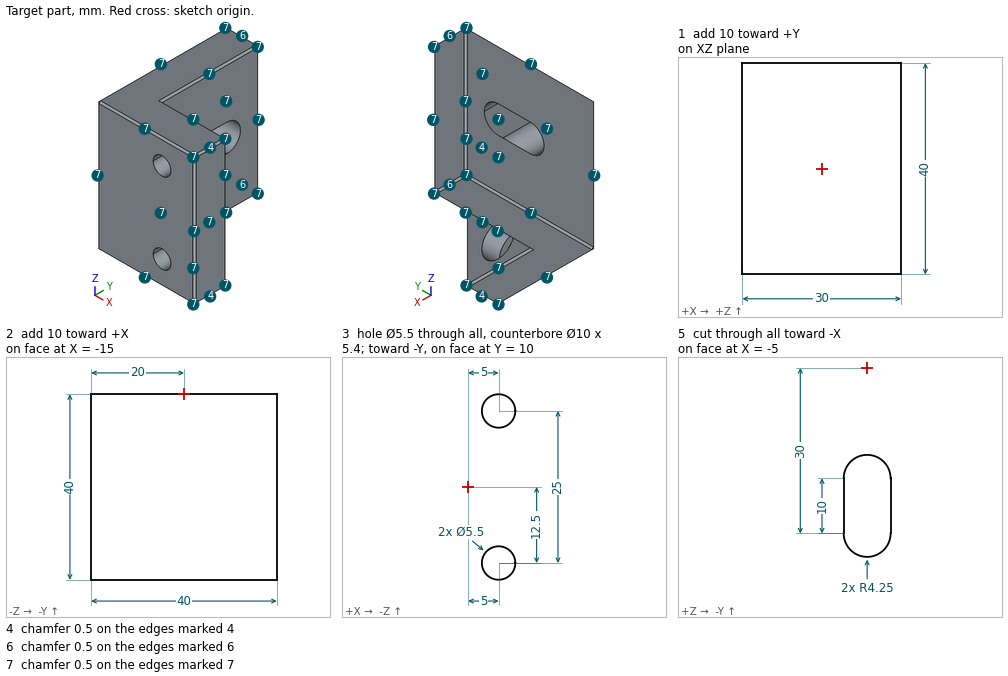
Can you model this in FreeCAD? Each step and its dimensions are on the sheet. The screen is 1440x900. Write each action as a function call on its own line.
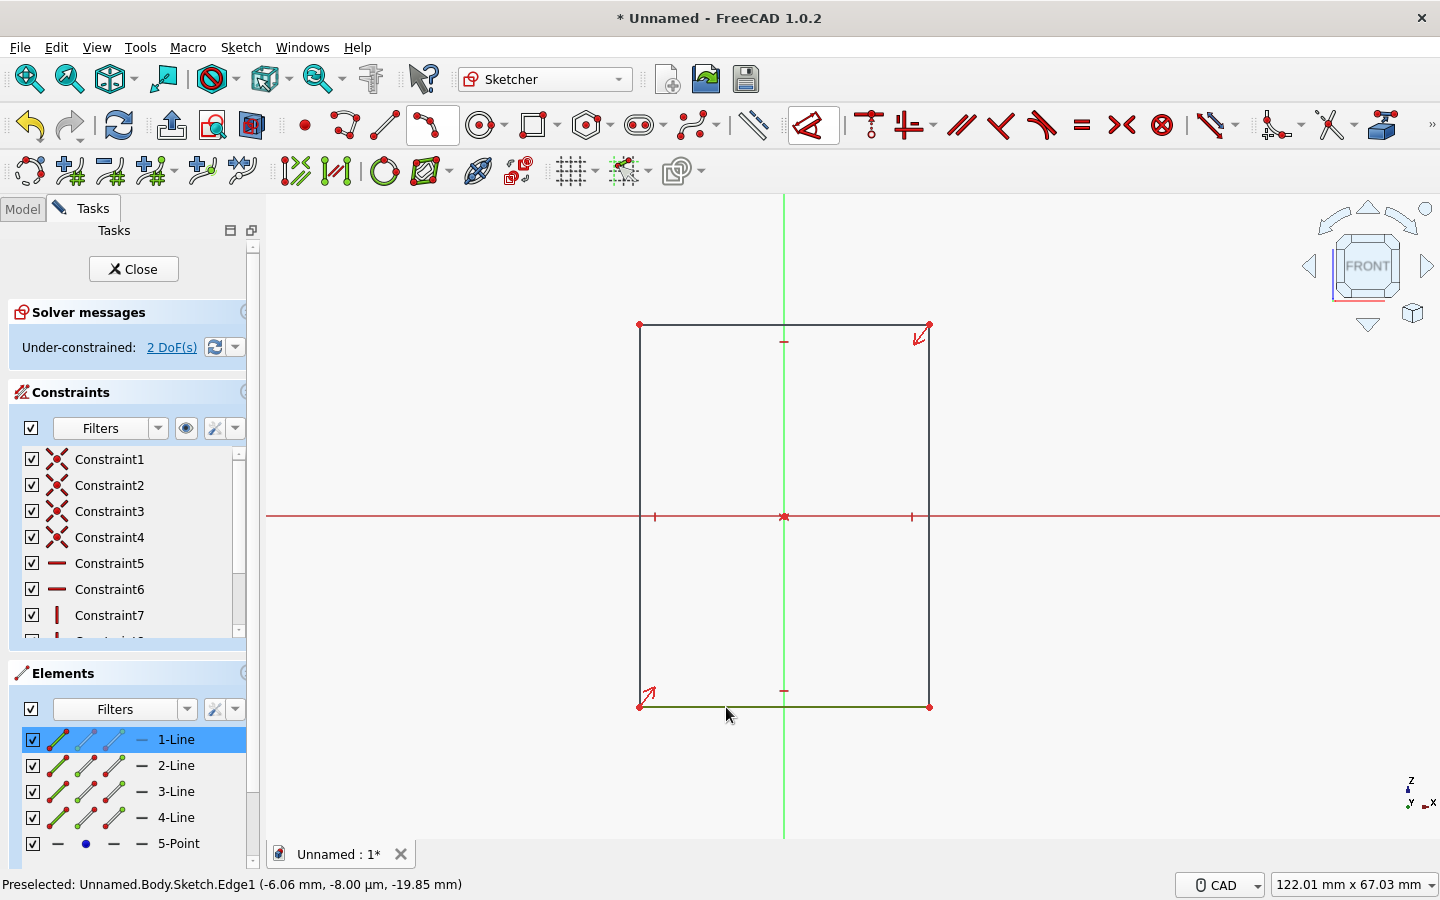
click(834, 126)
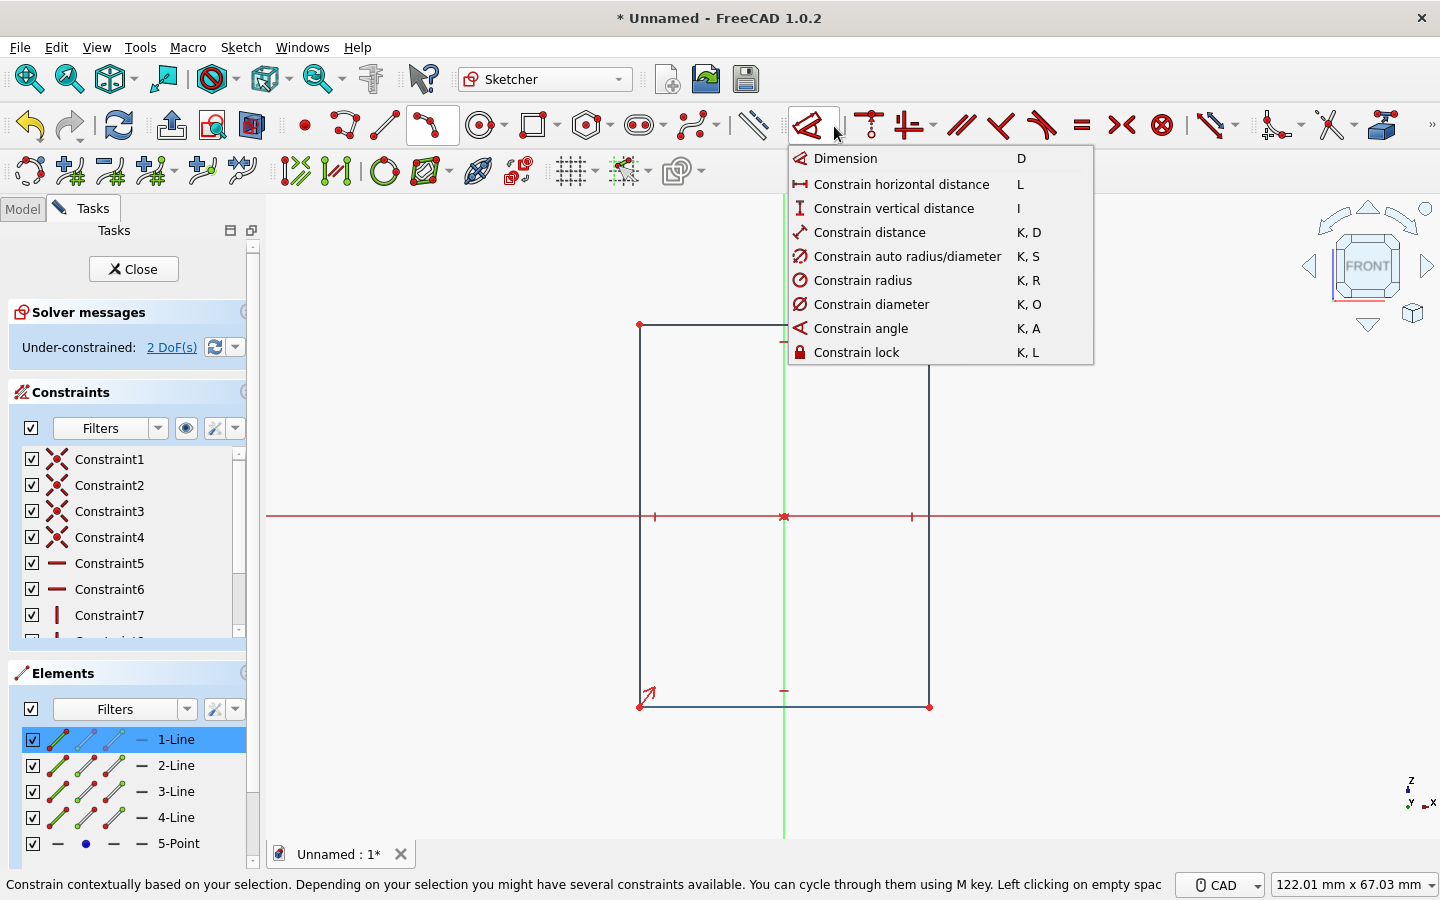
click(941, 184)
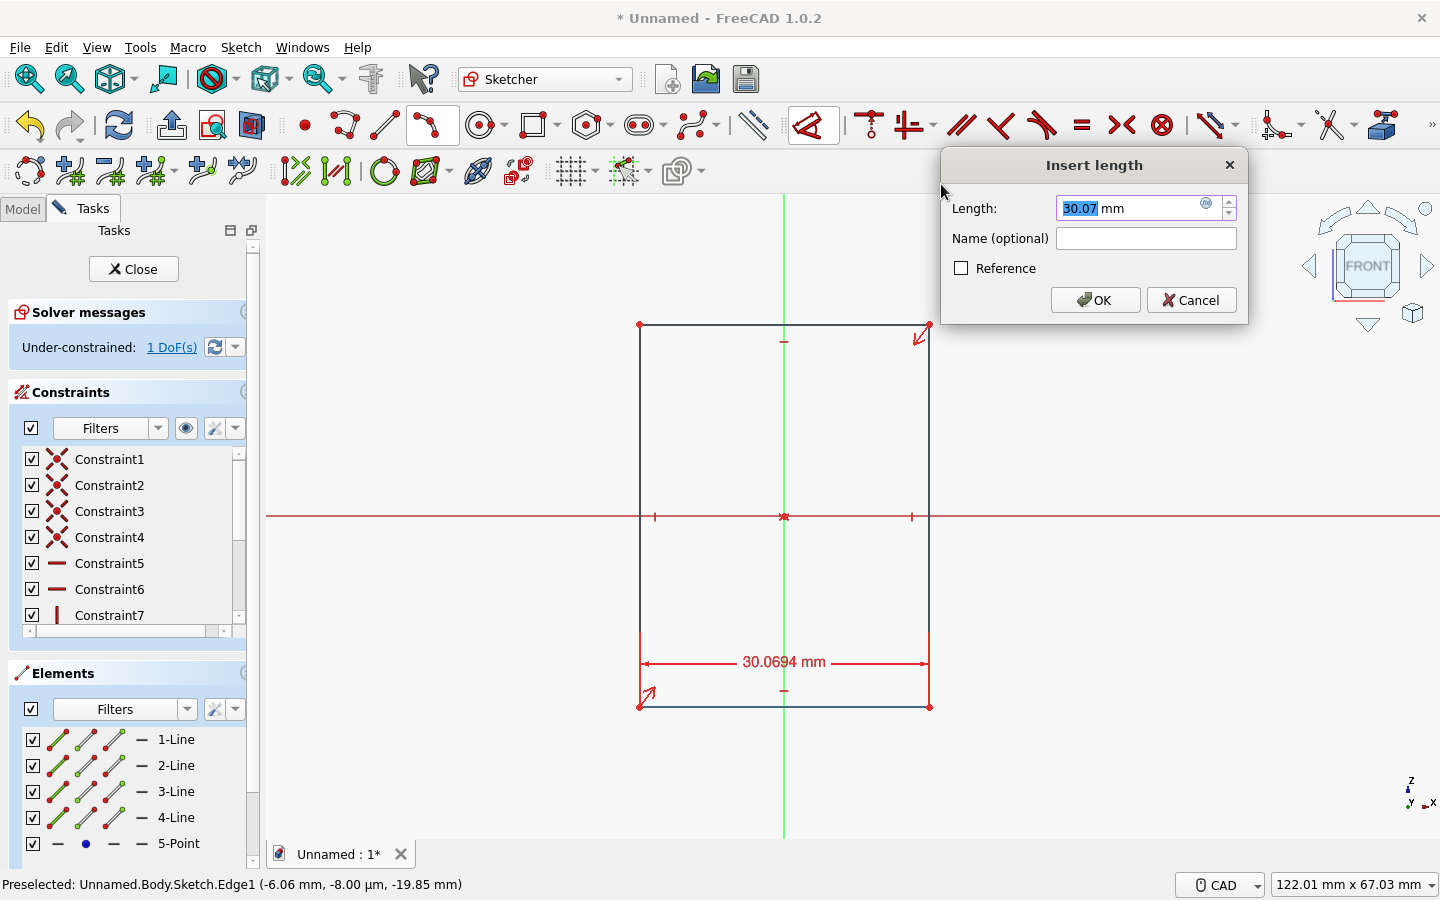
text(30)
key(Return)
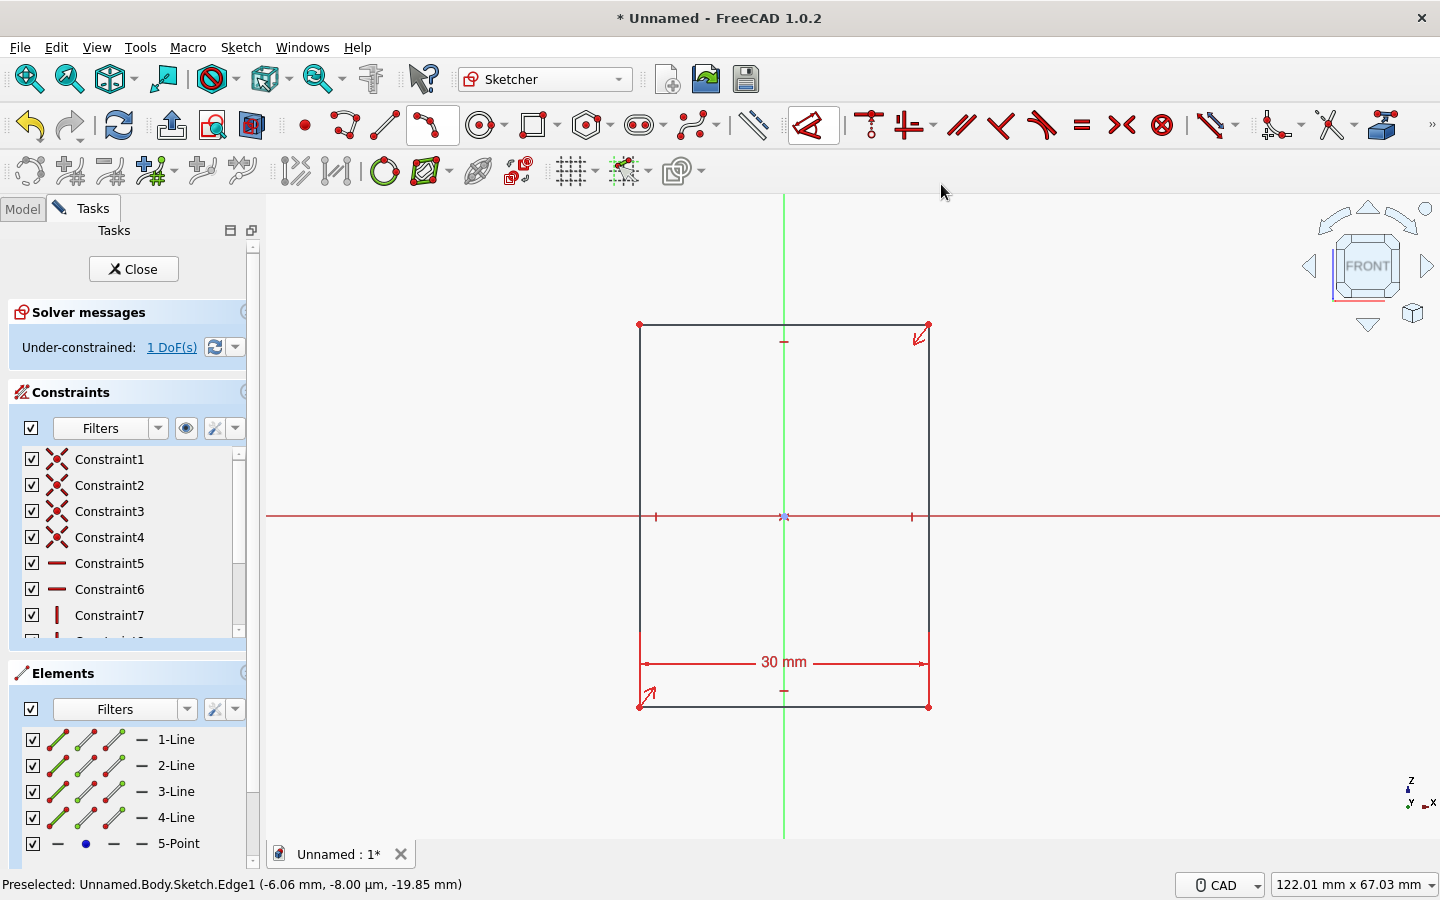
click(929, 592)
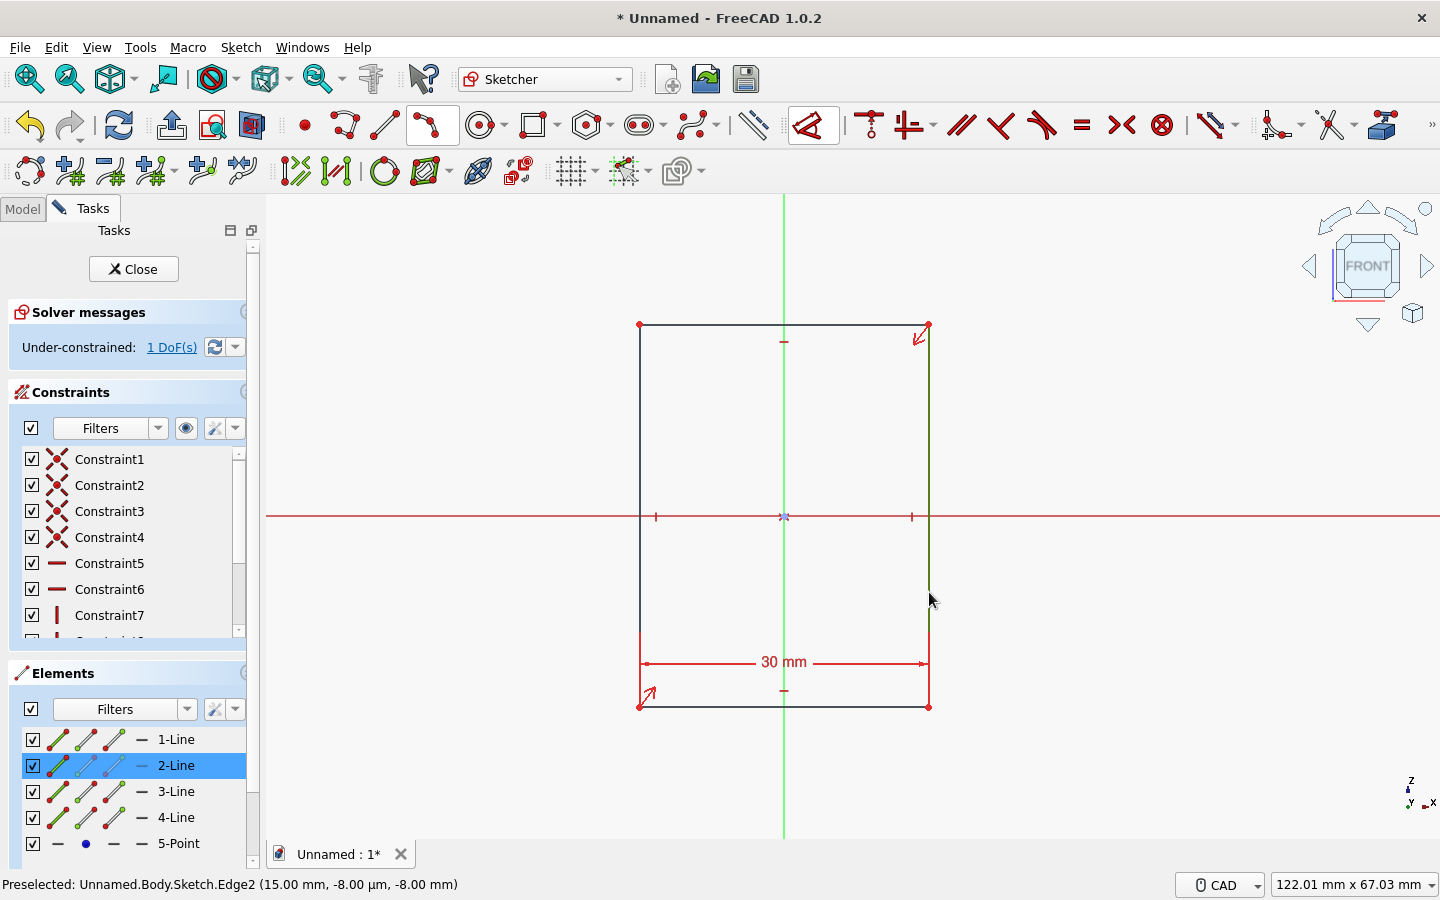
key(i)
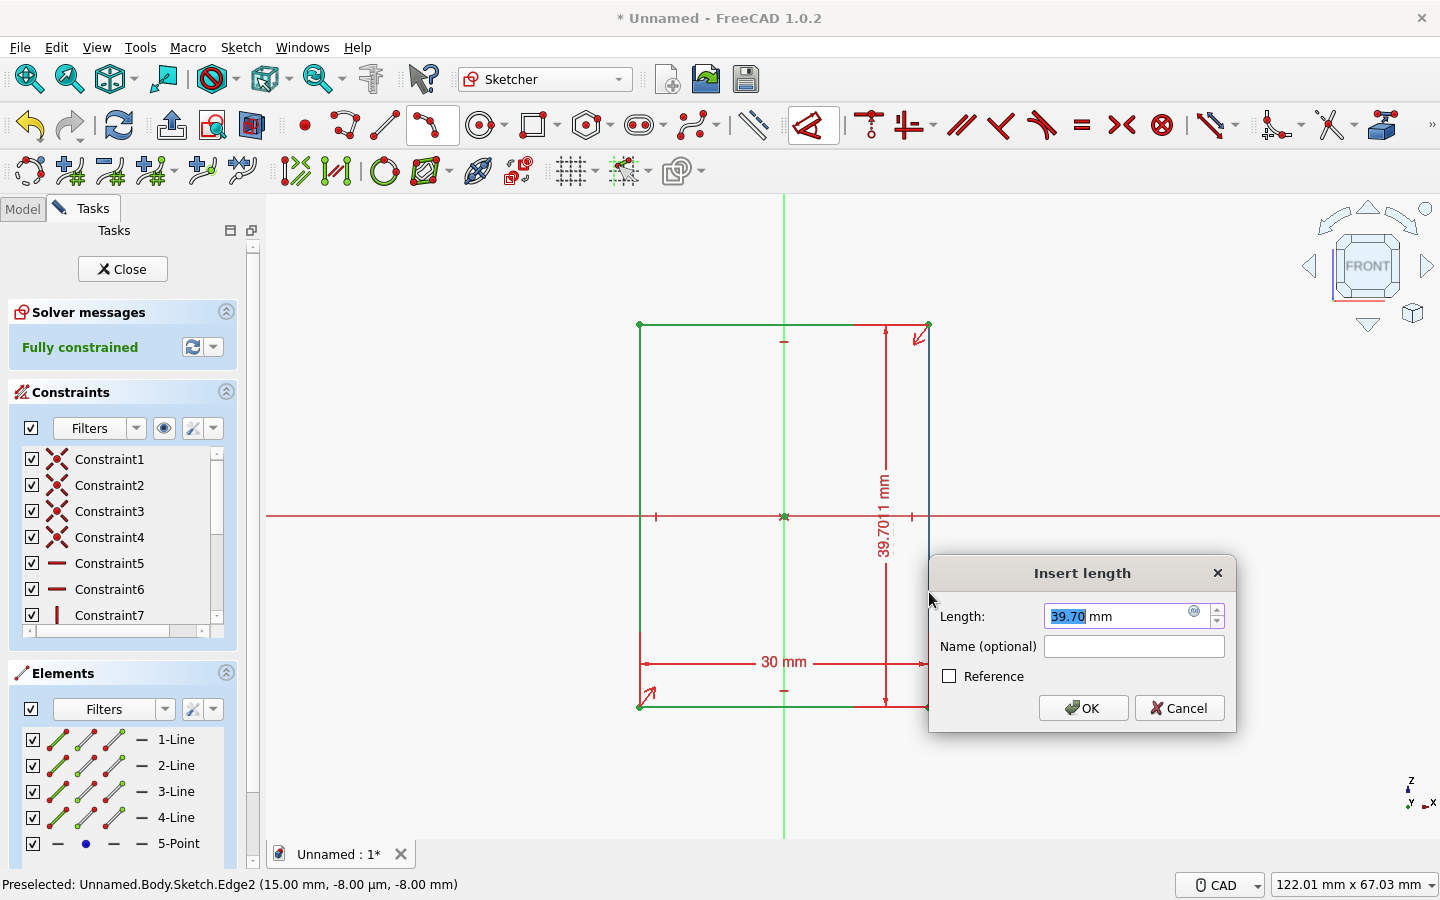
text(40)
key(Return)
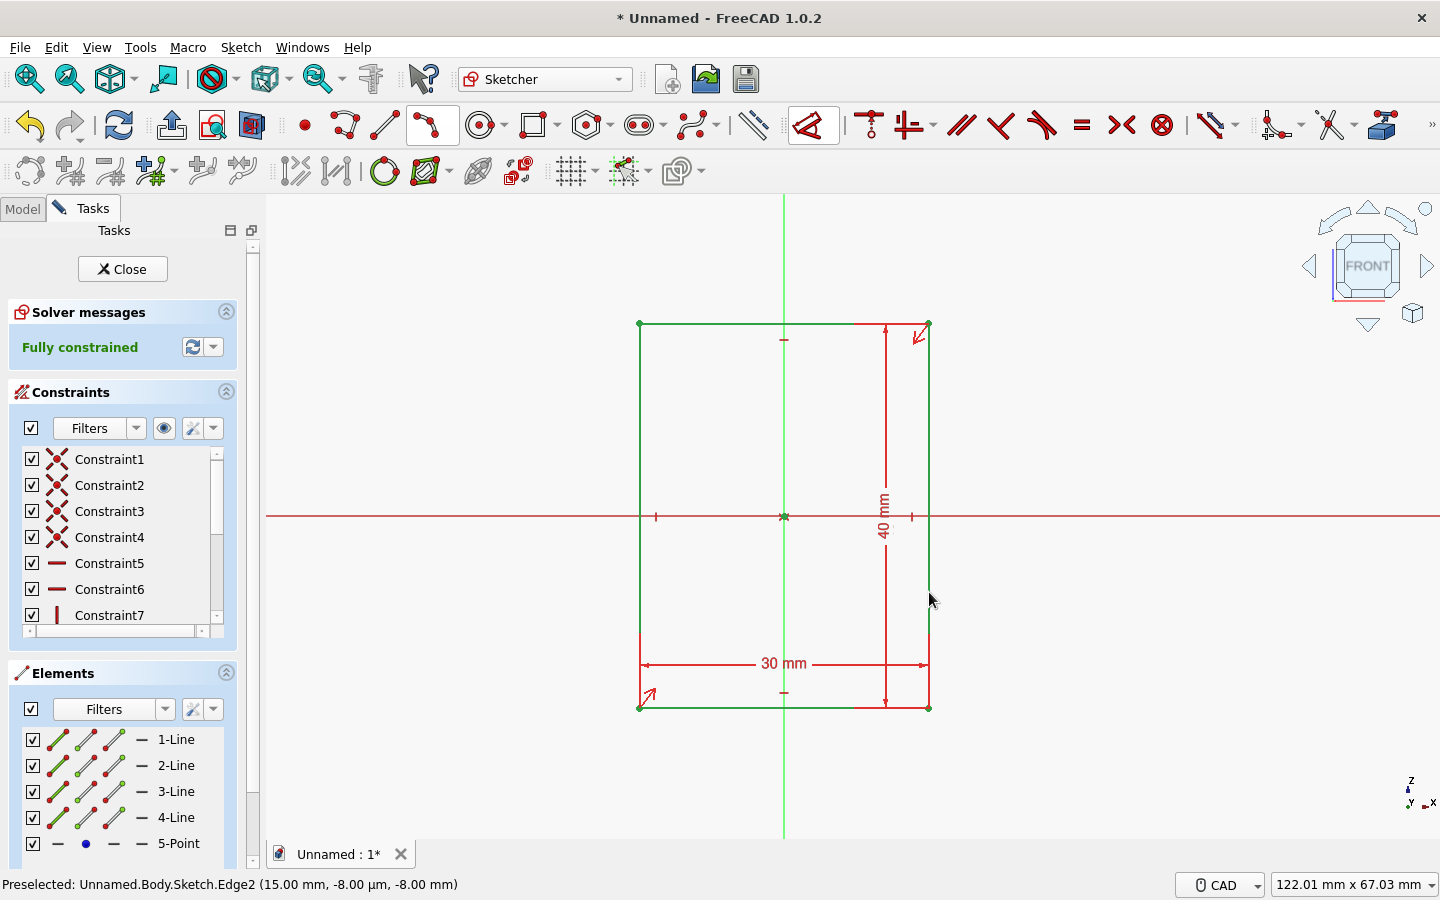
click(123, 269)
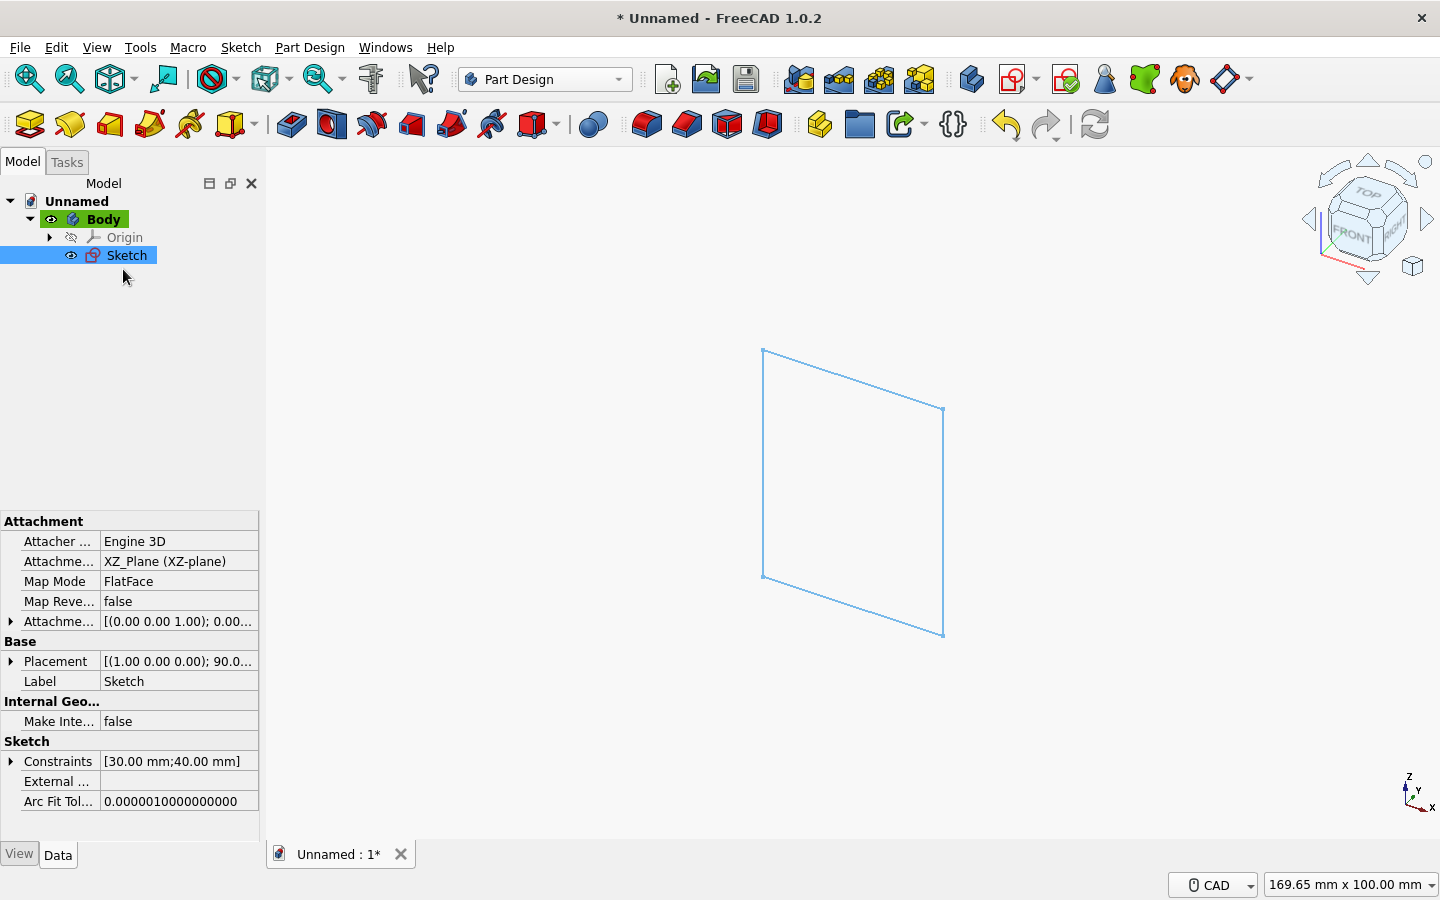
click(30, 124)